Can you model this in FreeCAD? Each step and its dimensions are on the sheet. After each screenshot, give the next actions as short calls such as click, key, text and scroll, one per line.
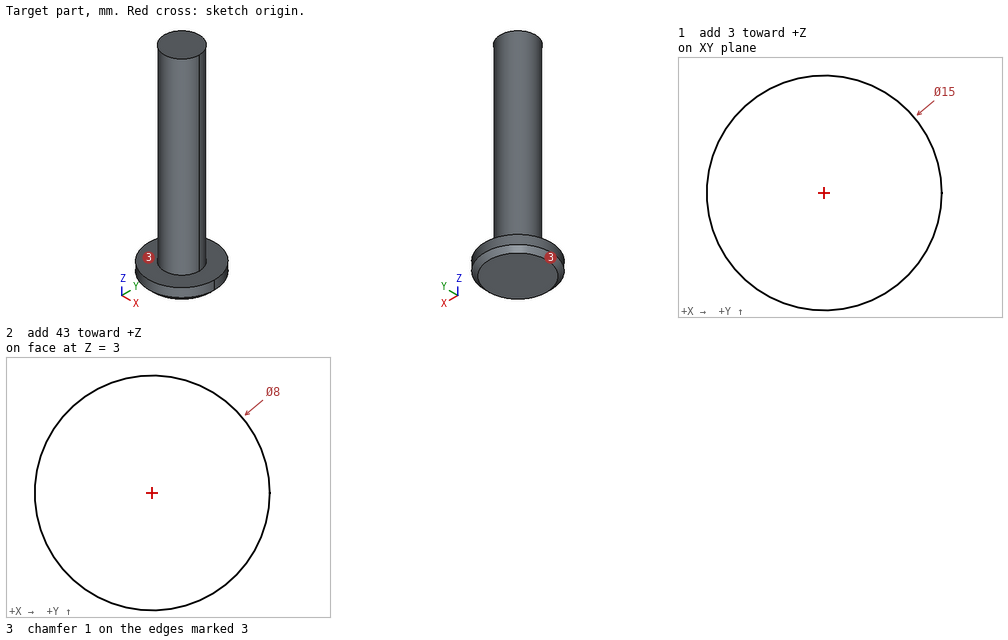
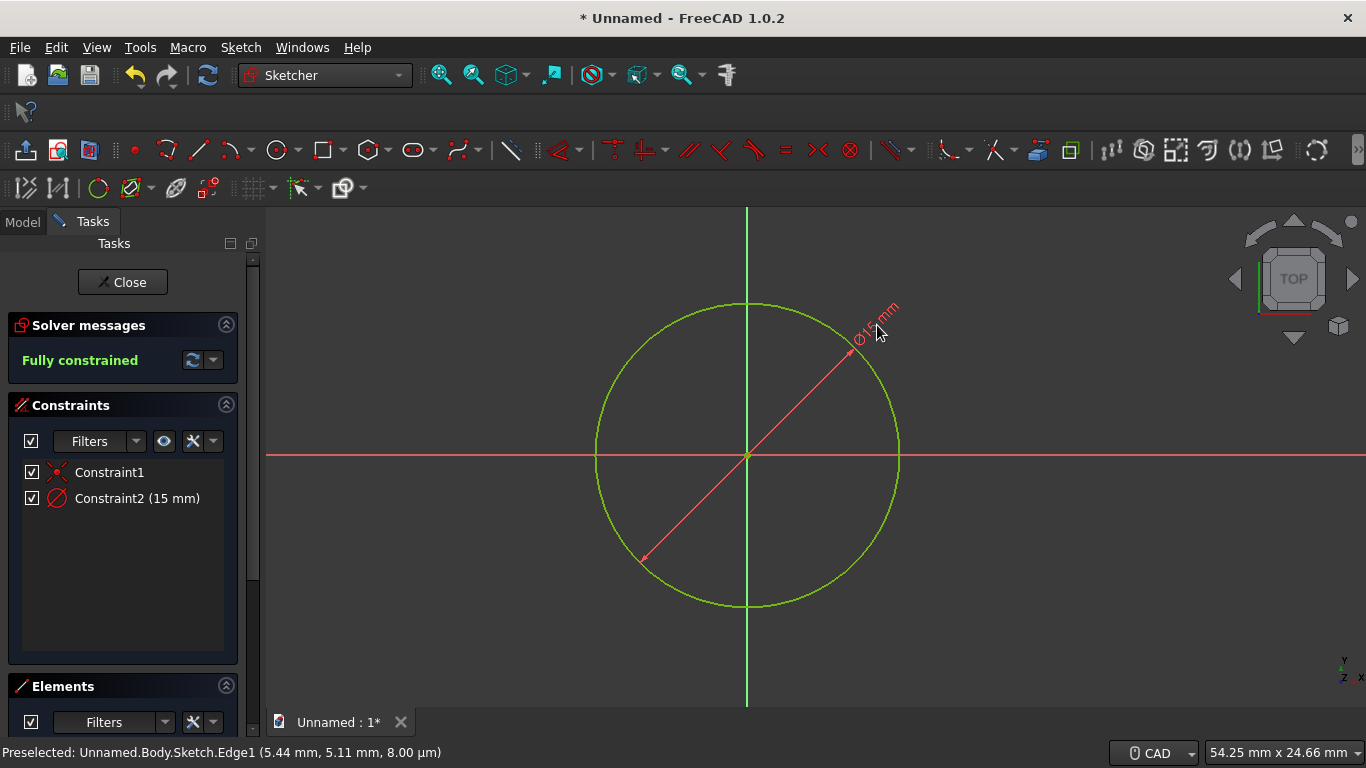
click(123, 282)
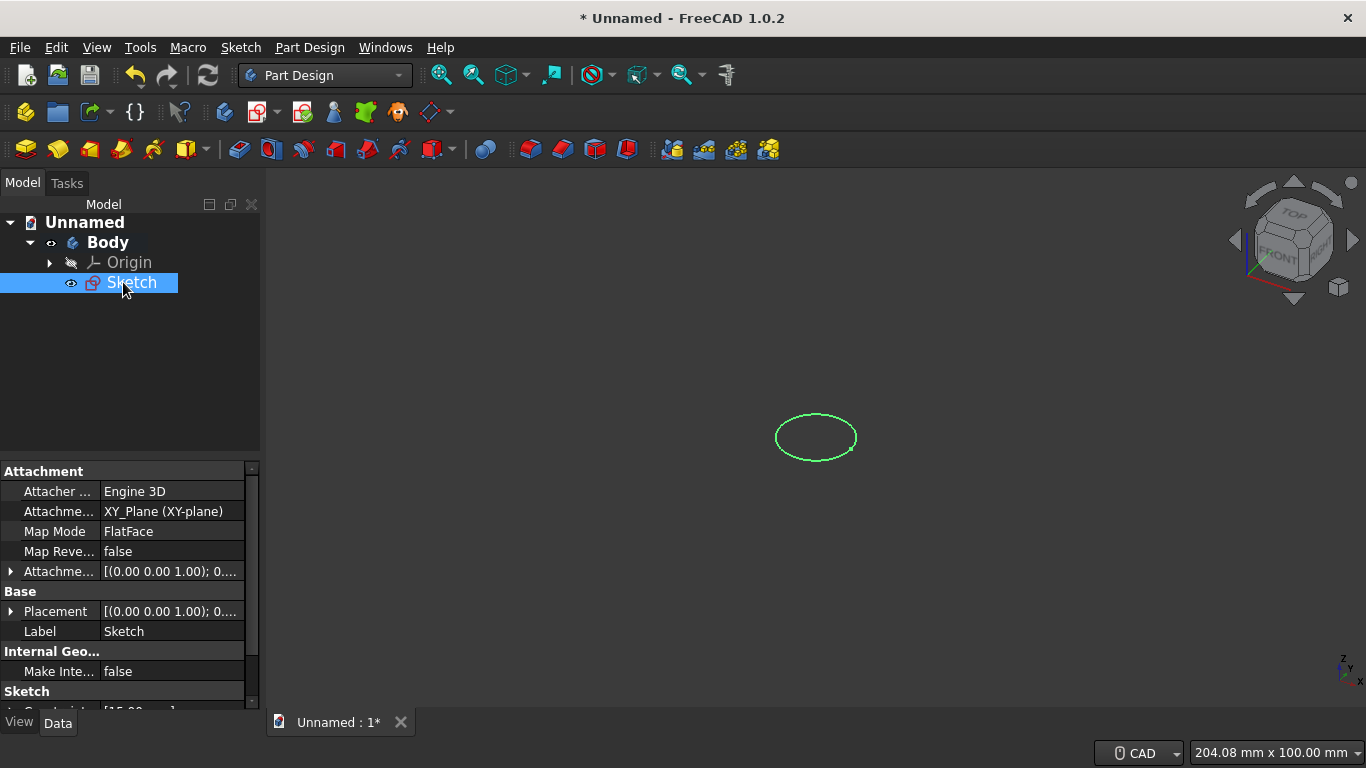
click(26, 150)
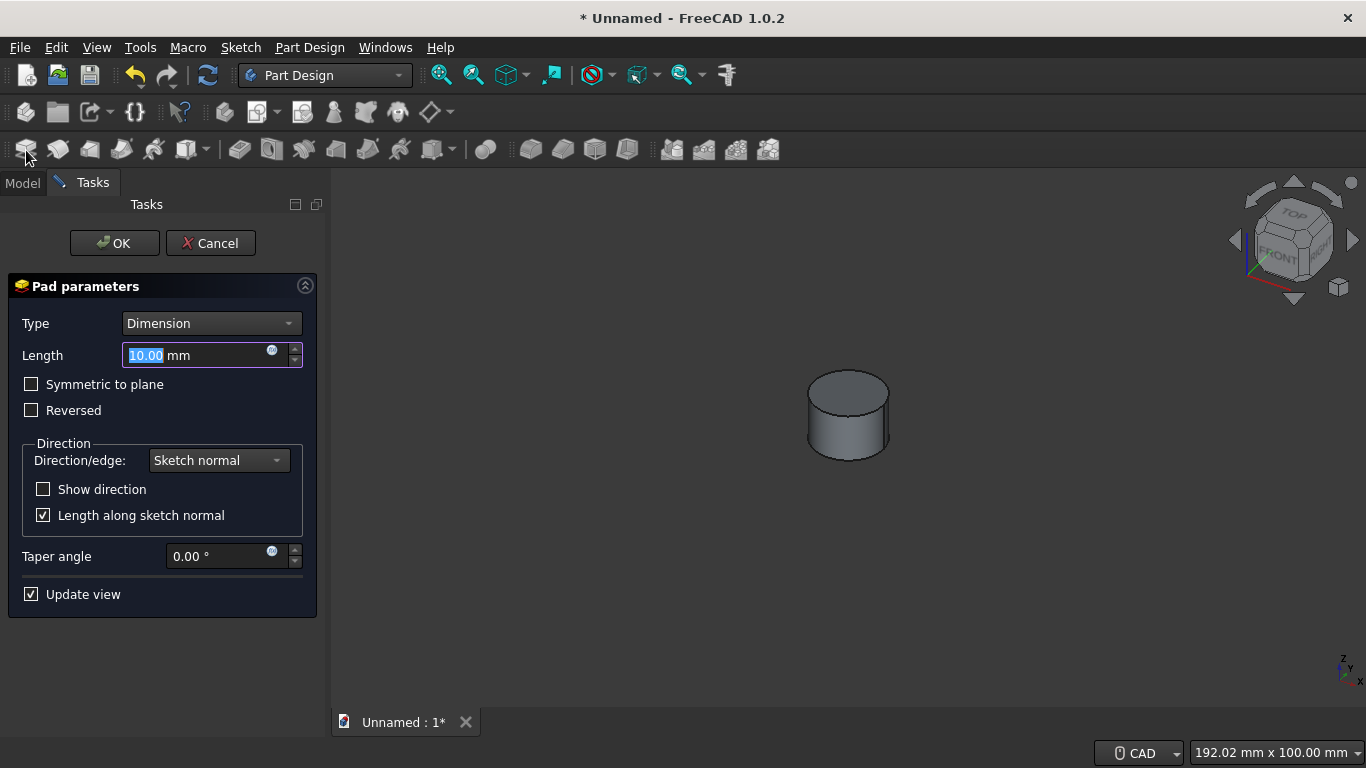
text(3)
key(Tab)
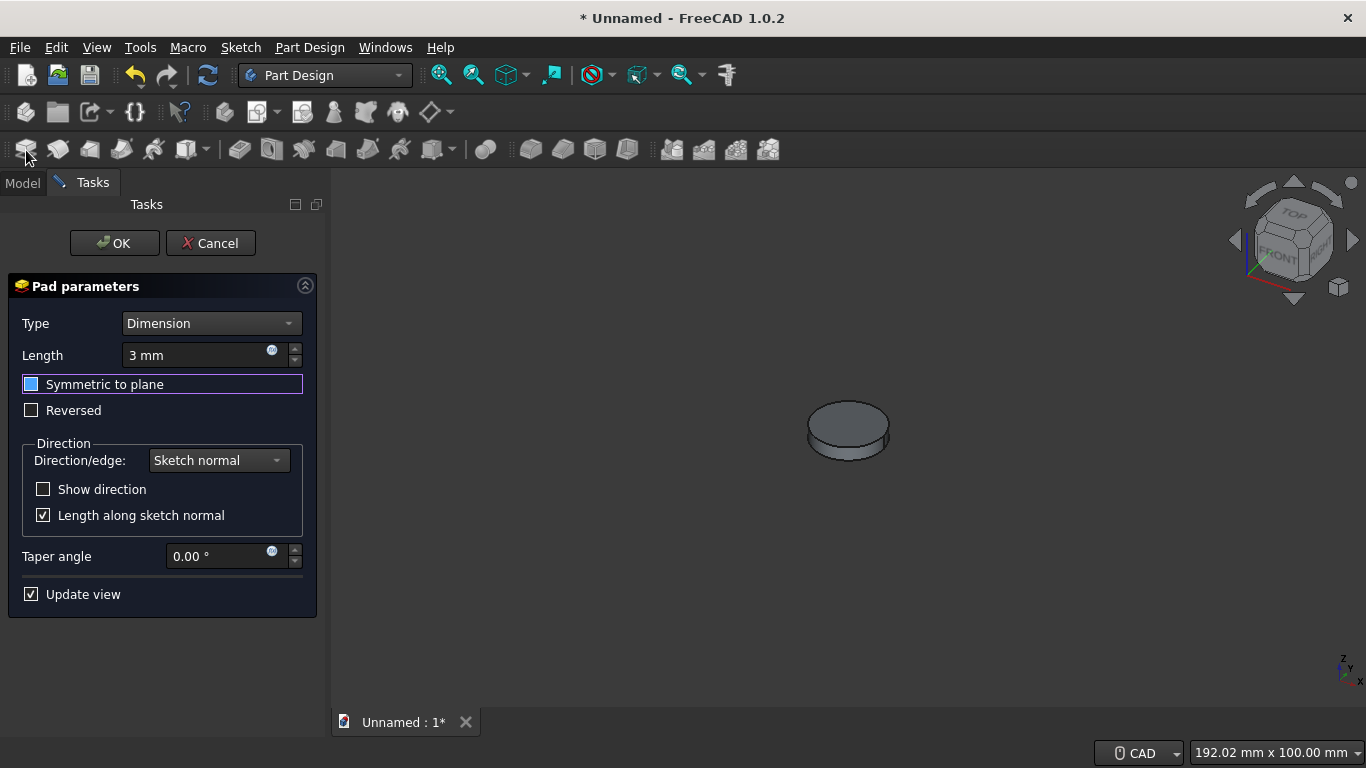
click(115, 243)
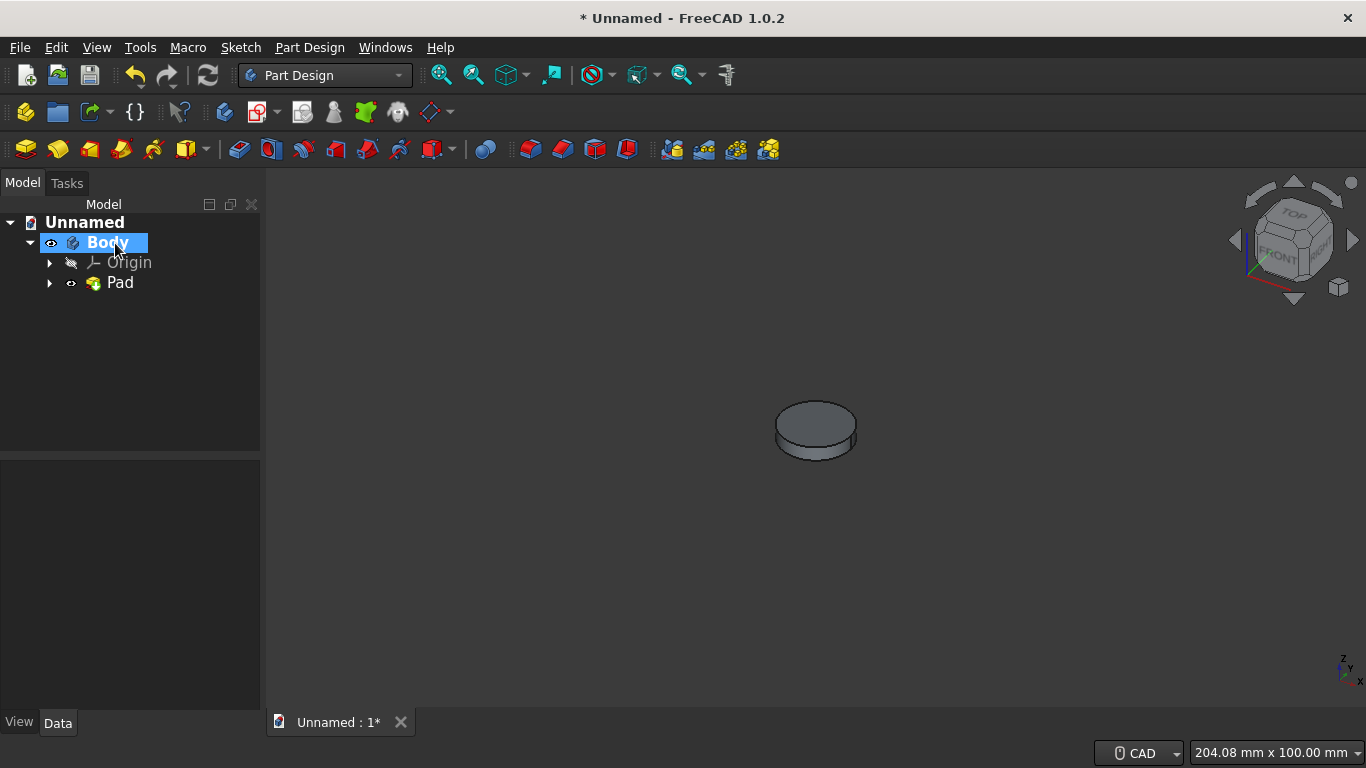
click(442, 76)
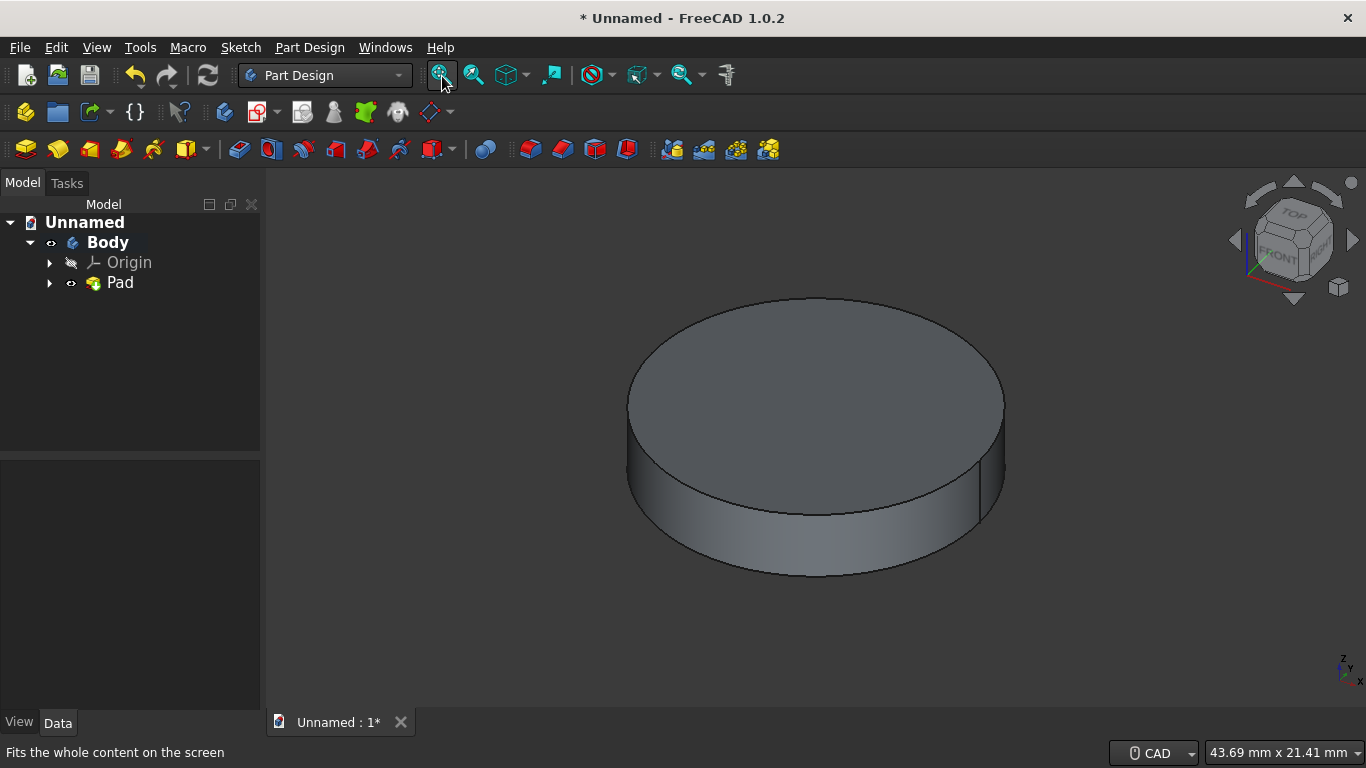
click(816, 406)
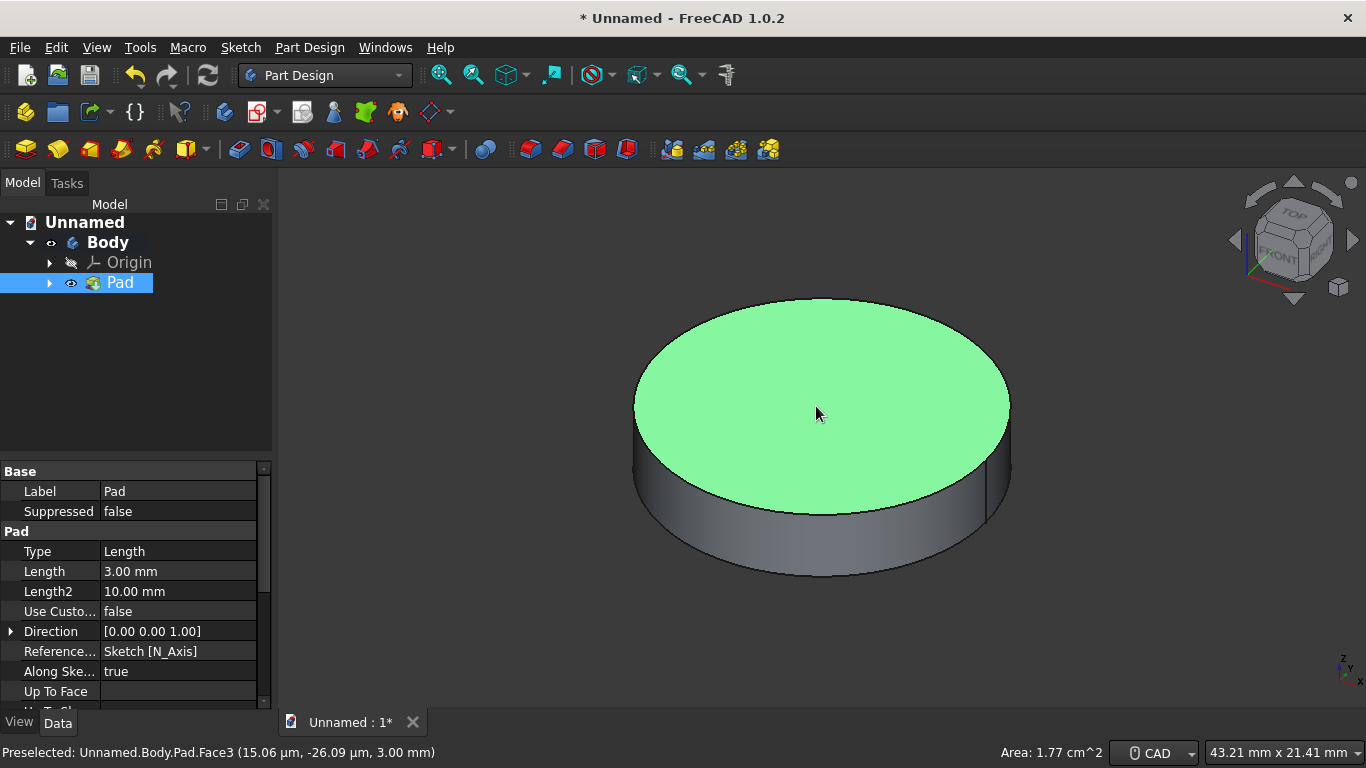
click(258, 112)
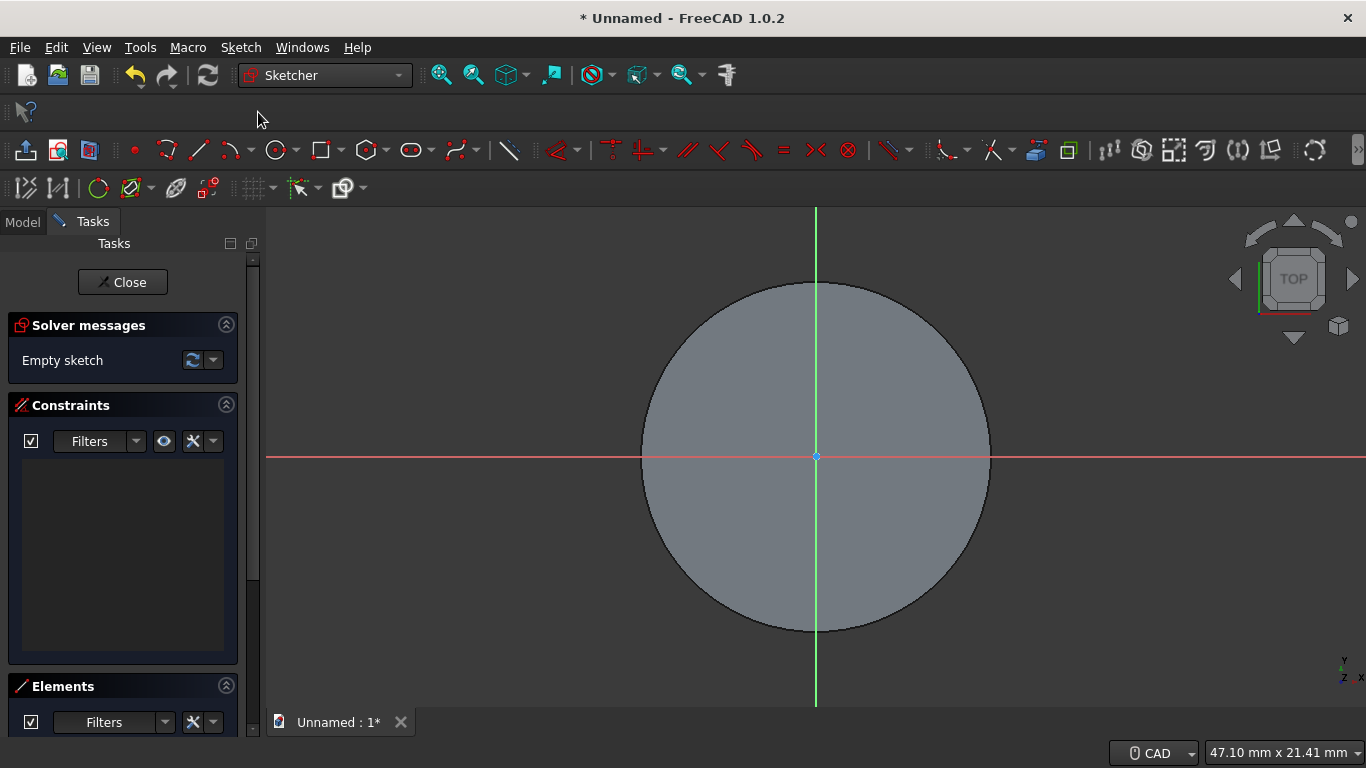
scroll(899, 457, up, 3)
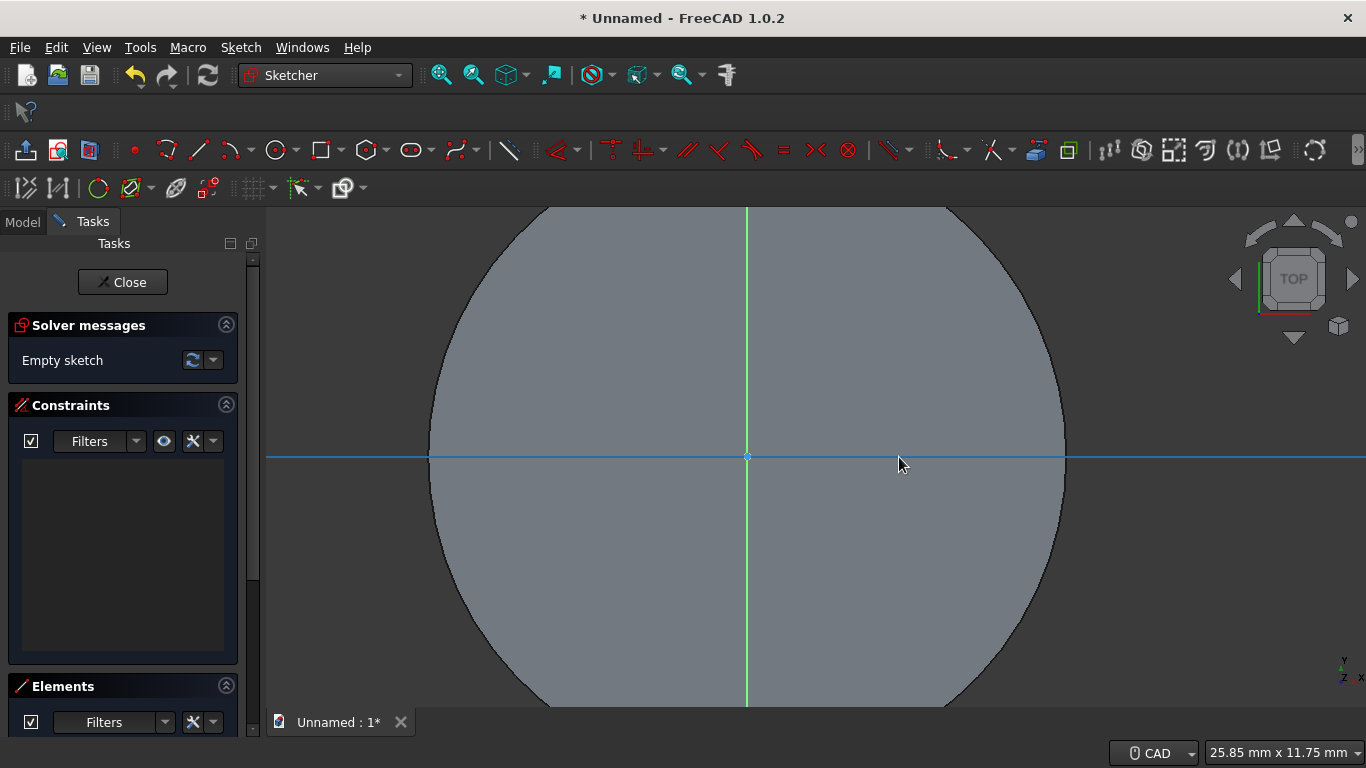
click(276, 150)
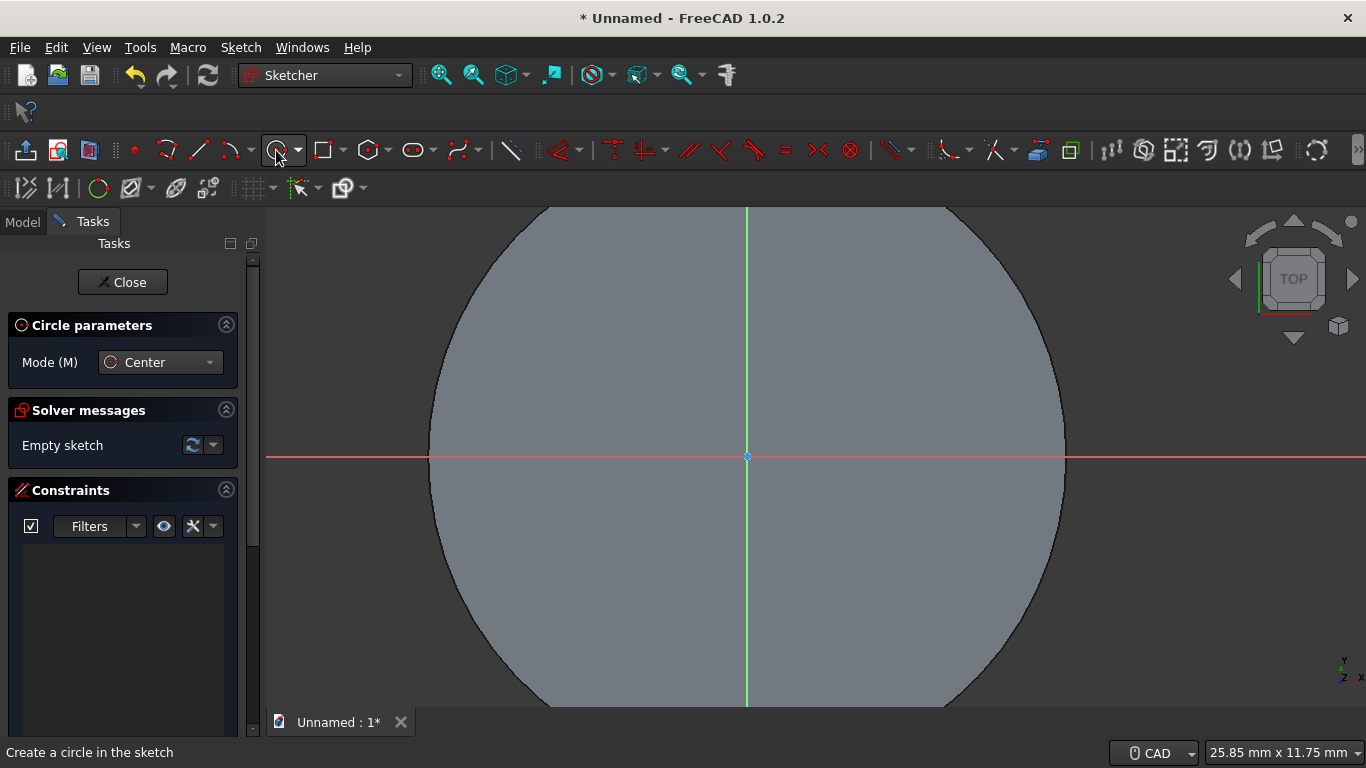
click(747, 457)
click(868, 336)
key(Escape)